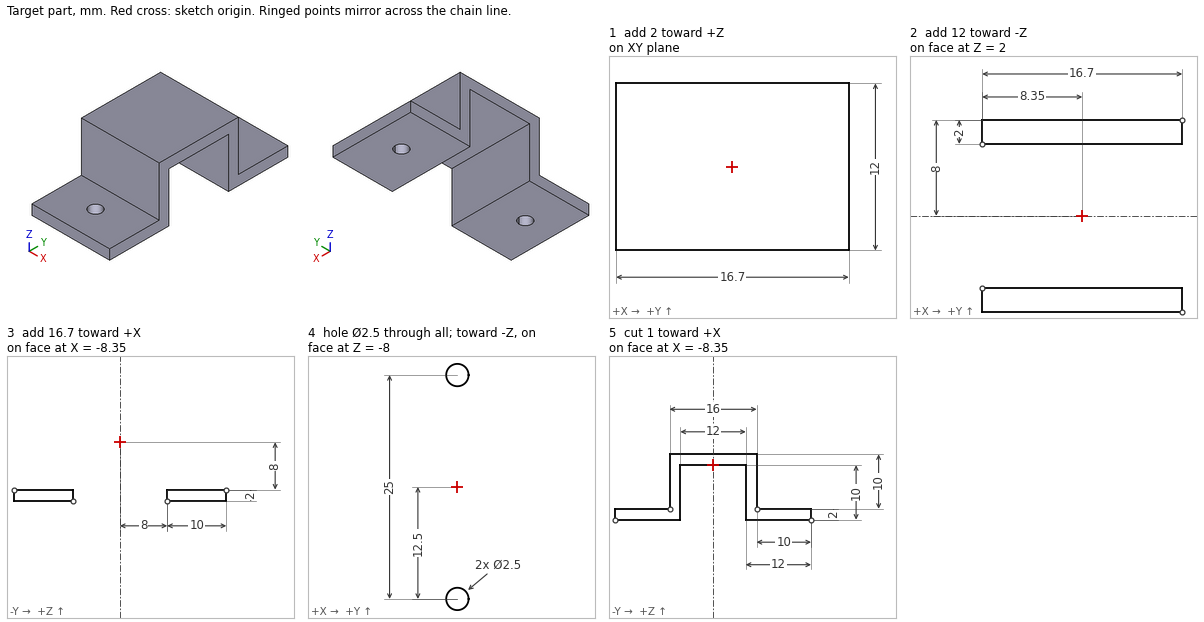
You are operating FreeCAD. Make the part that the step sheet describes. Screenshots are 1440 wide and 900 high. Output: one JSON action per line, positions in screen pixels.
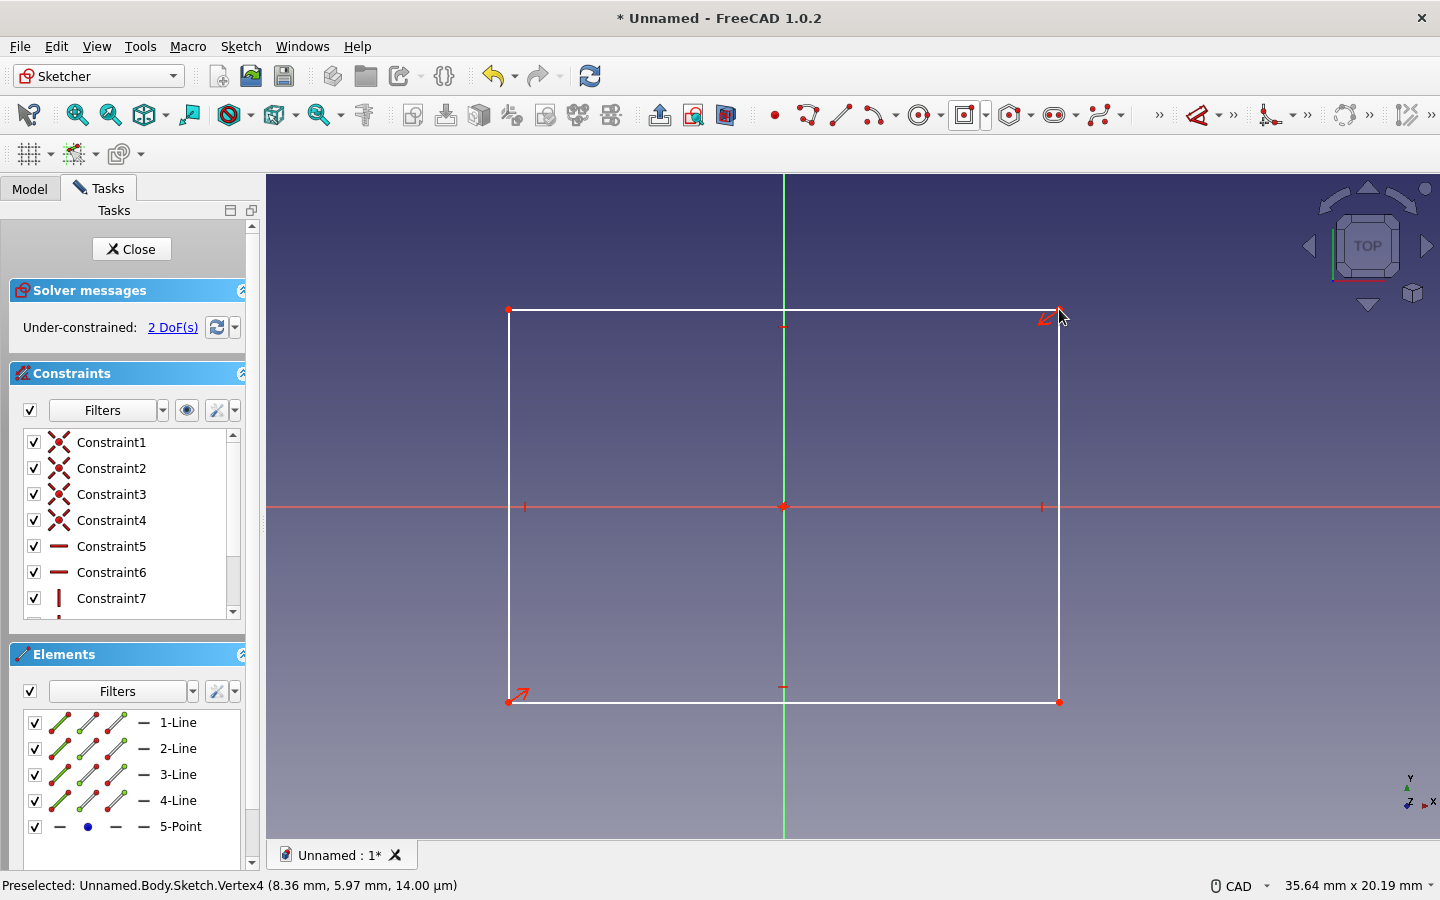
{"action": "left_click", "coordinate": [1196, 116]}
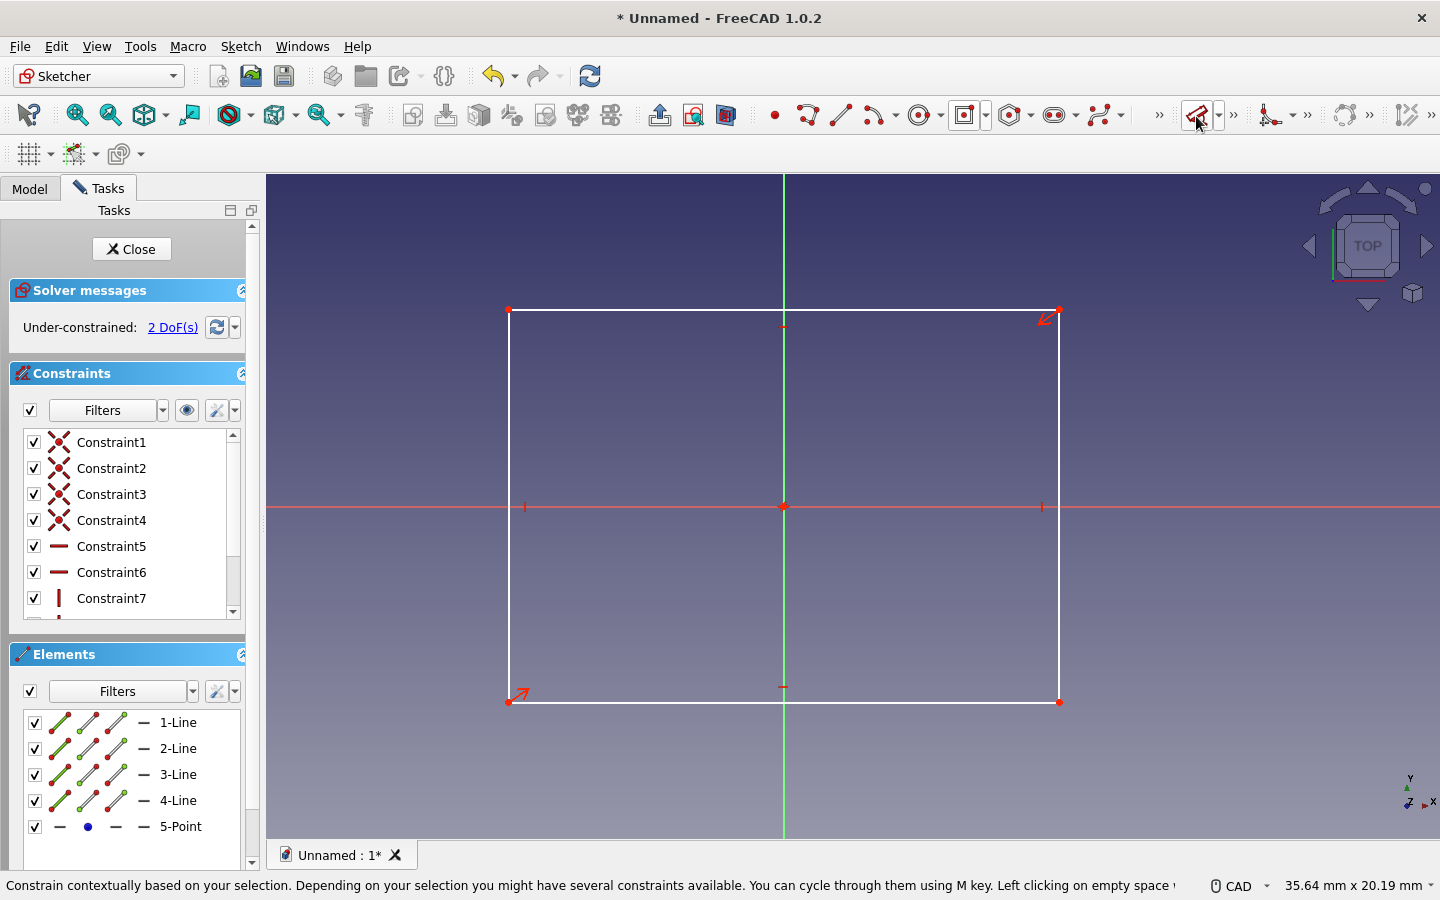
{"action": "left_click", "coordinate": [1059, 585]}
{"action": "left_click", "coordinate": [1093, 416]}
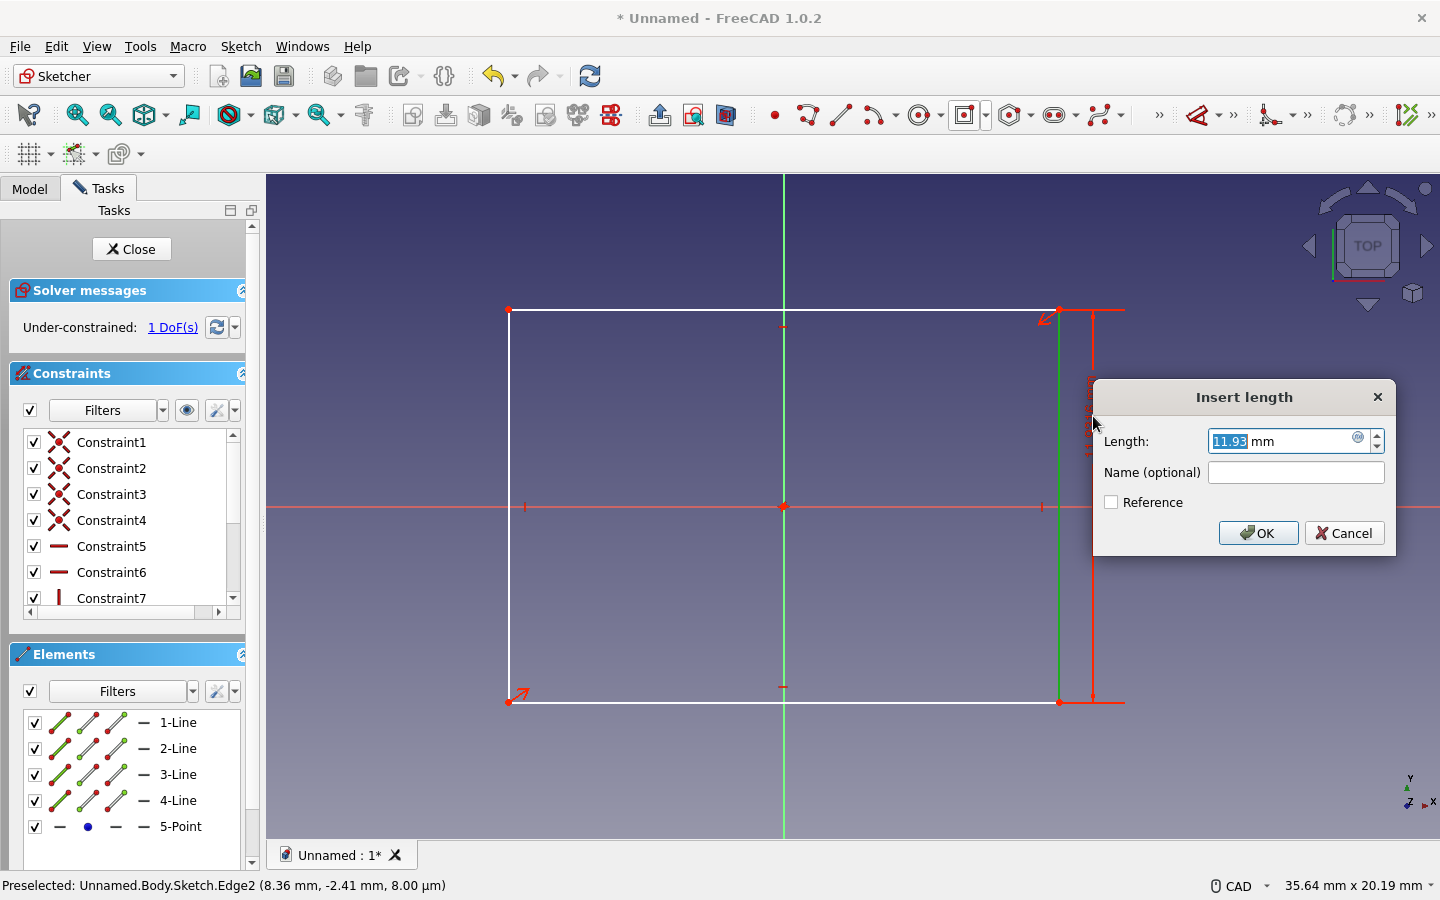
{"action": "type", "text": "12"}
{"action": "key", "text": "Return"}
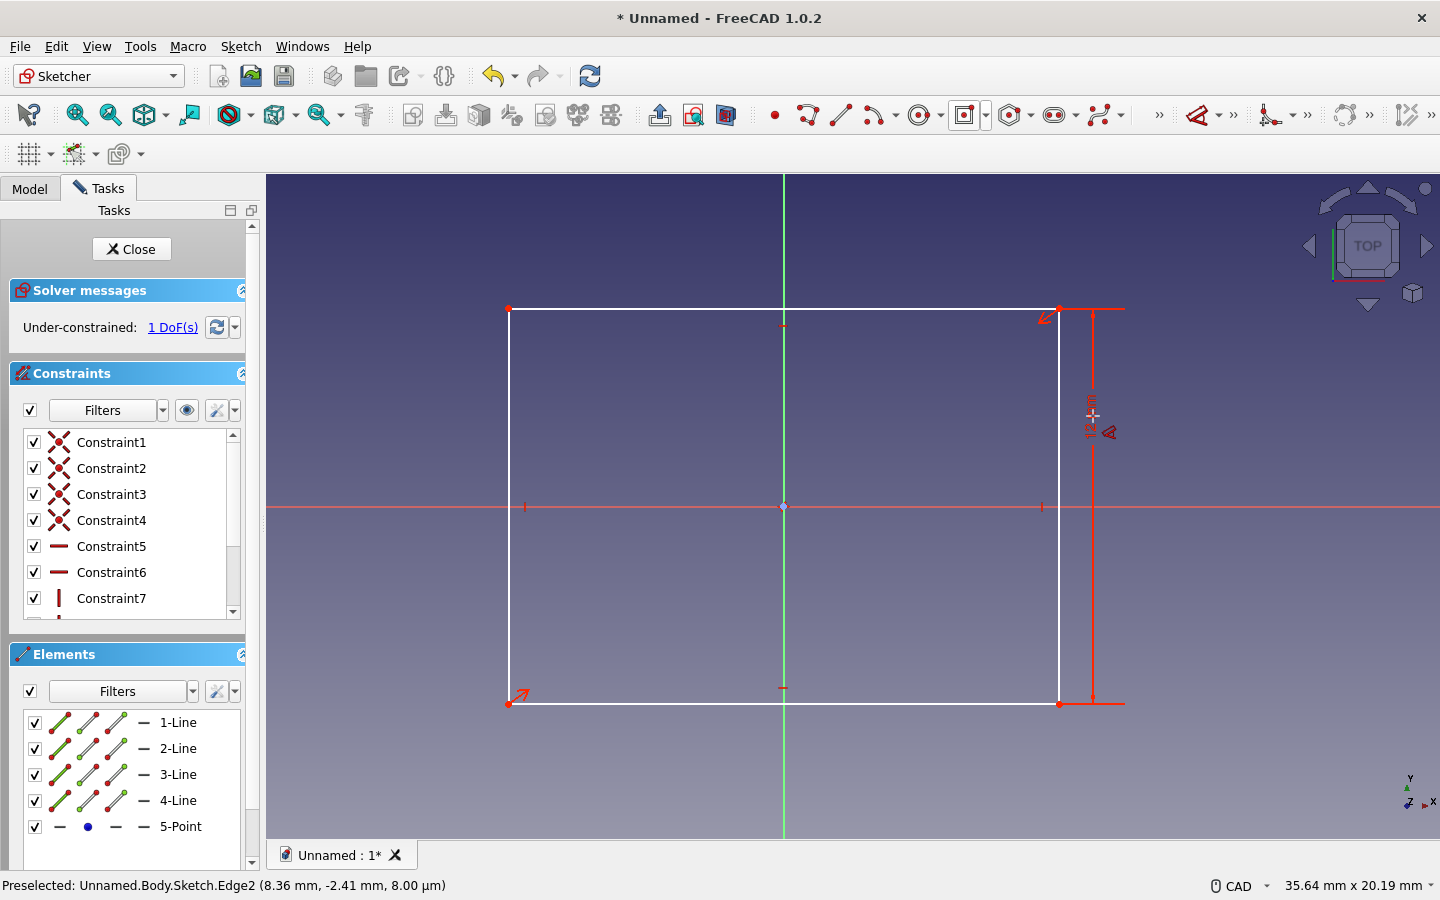
{"action": "left_click", "coordinate": [674, 704]}
{"action": "left_click", "coordinate": [657, 738]}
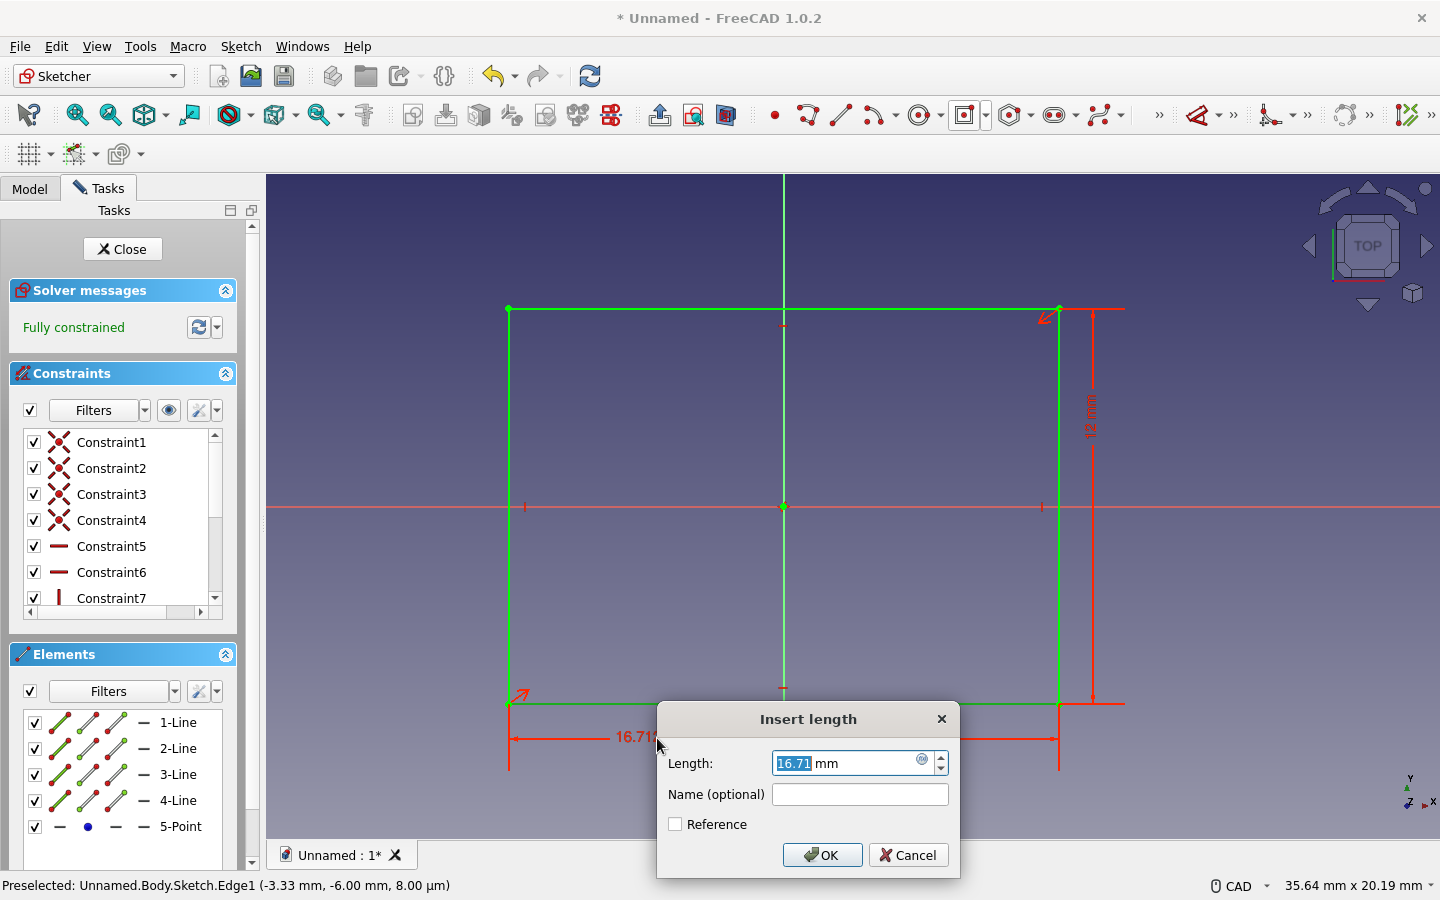
{"action": "type", "text": "16.7"}
{"action": "key", "text": "Return"}
{"action": "key", "text": "Escape"}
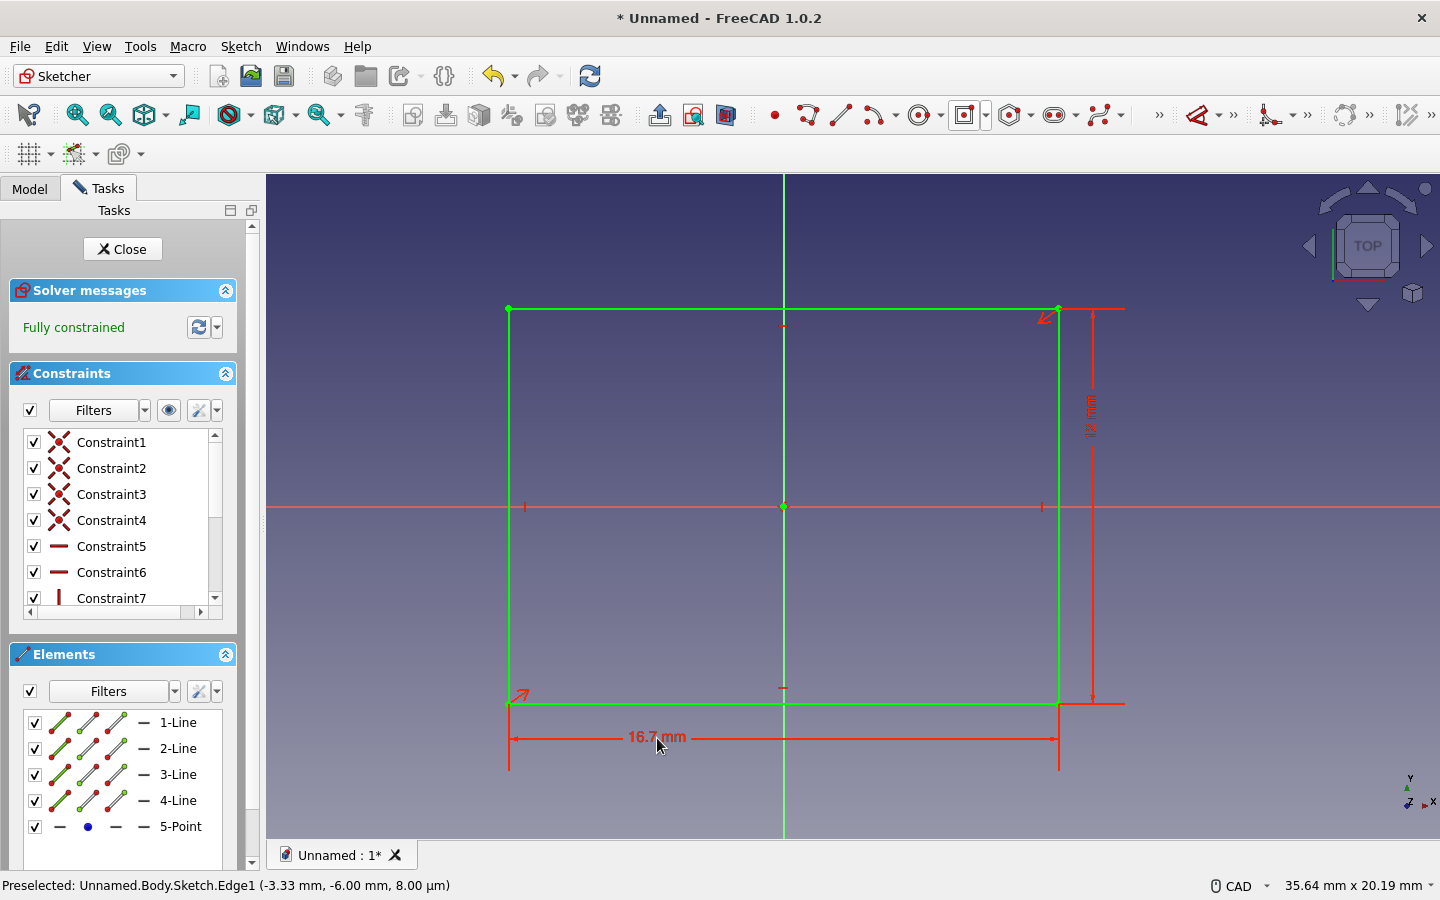
{"action": "left_click", "coordinate": [123, 249]}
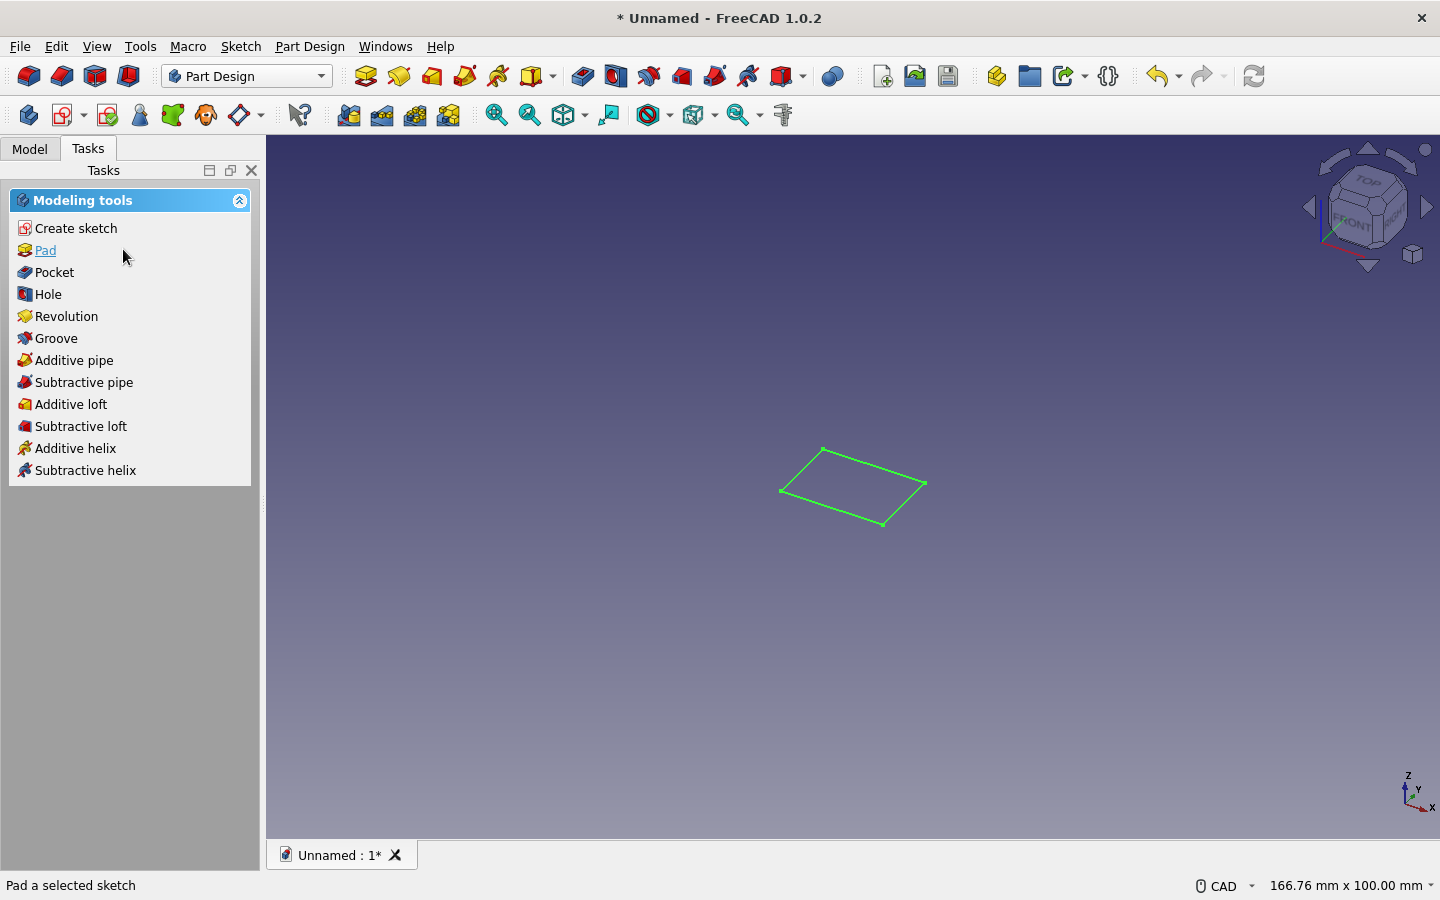
{"action": "left_click", "coordinate": [366, 76]}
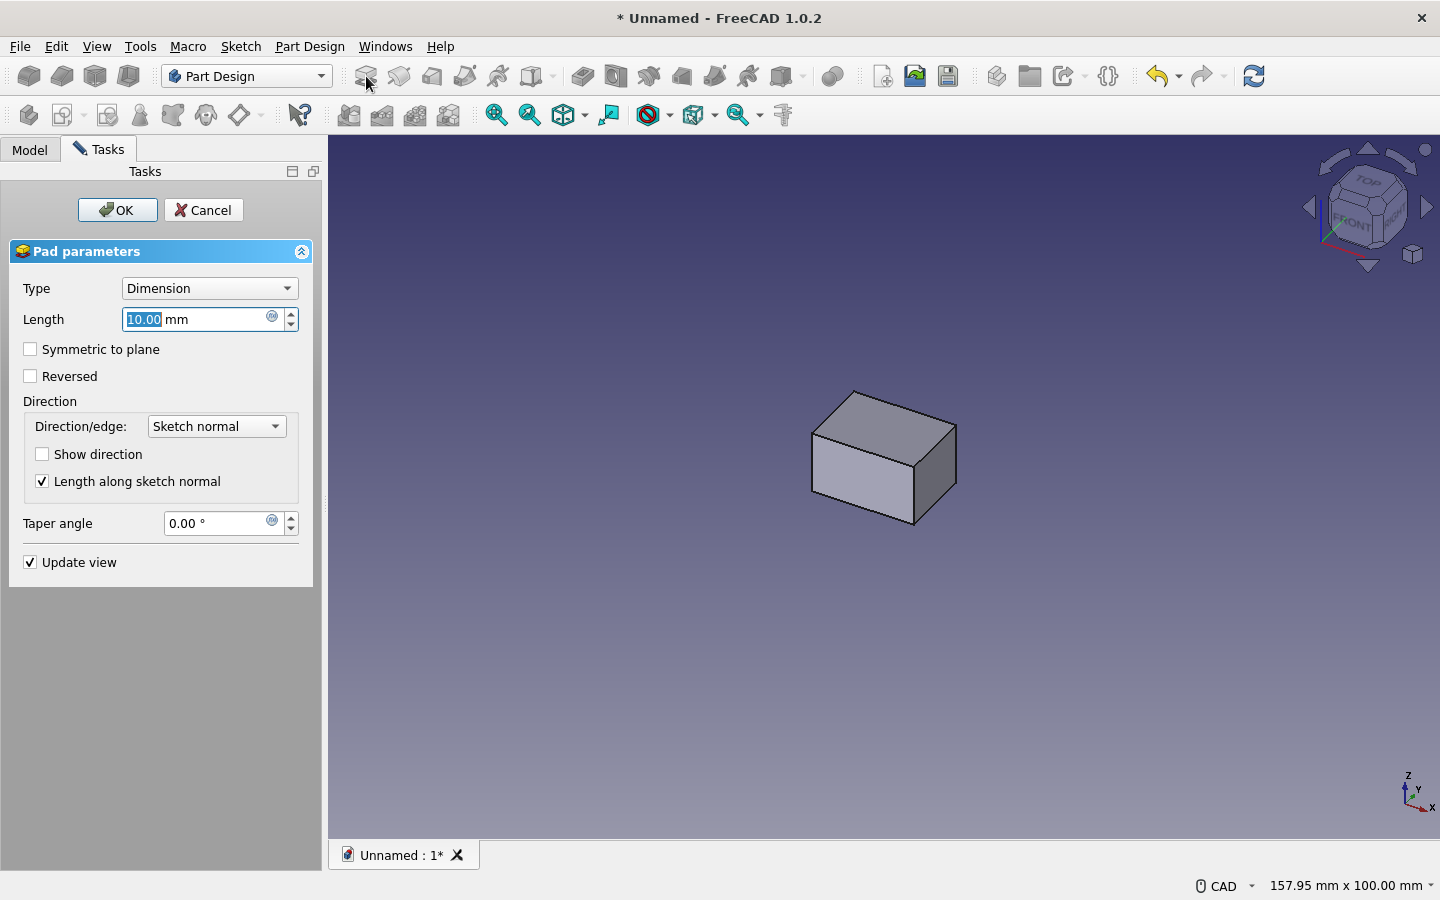
{"action": "type", "text": "2"}
{"action": "key", "text": "Tab"}